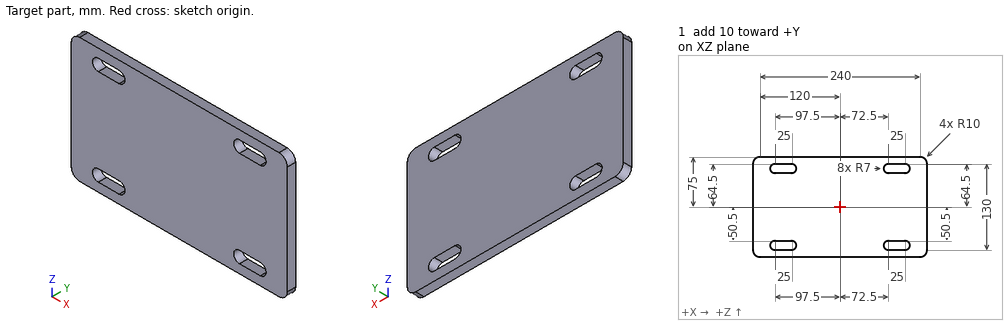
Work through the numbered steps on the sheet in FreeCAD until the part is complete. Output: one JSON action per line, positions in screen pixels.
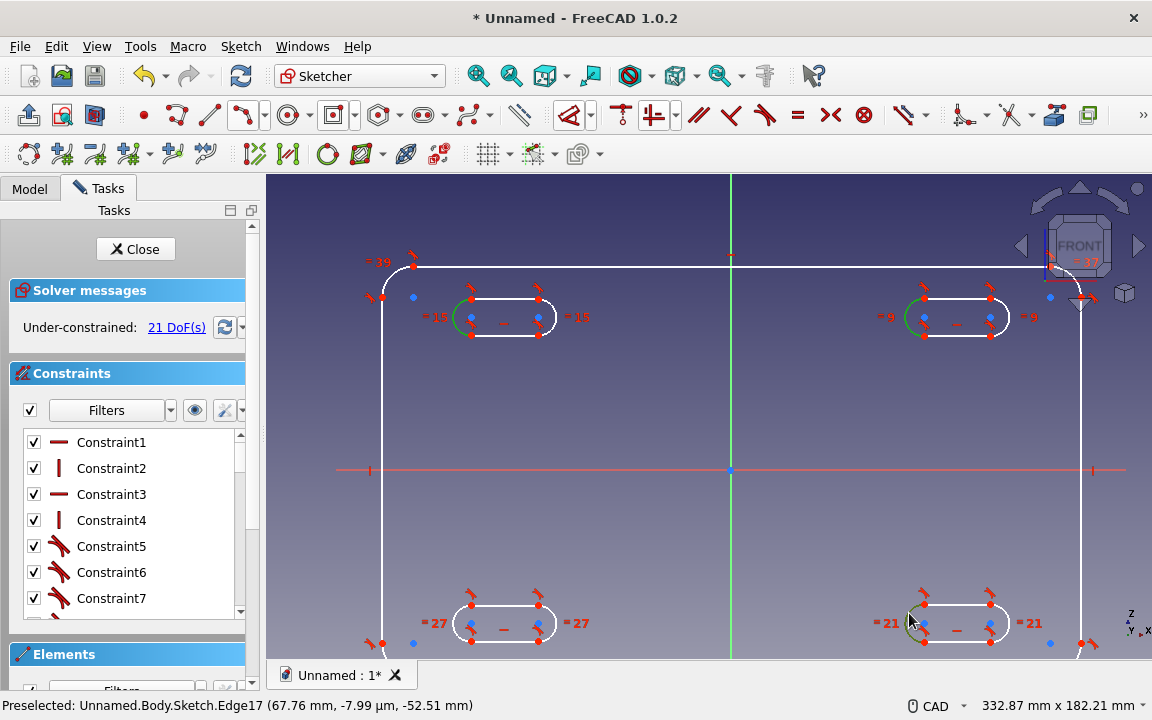
{"action": "left_click", "coordinate": [457, 613]}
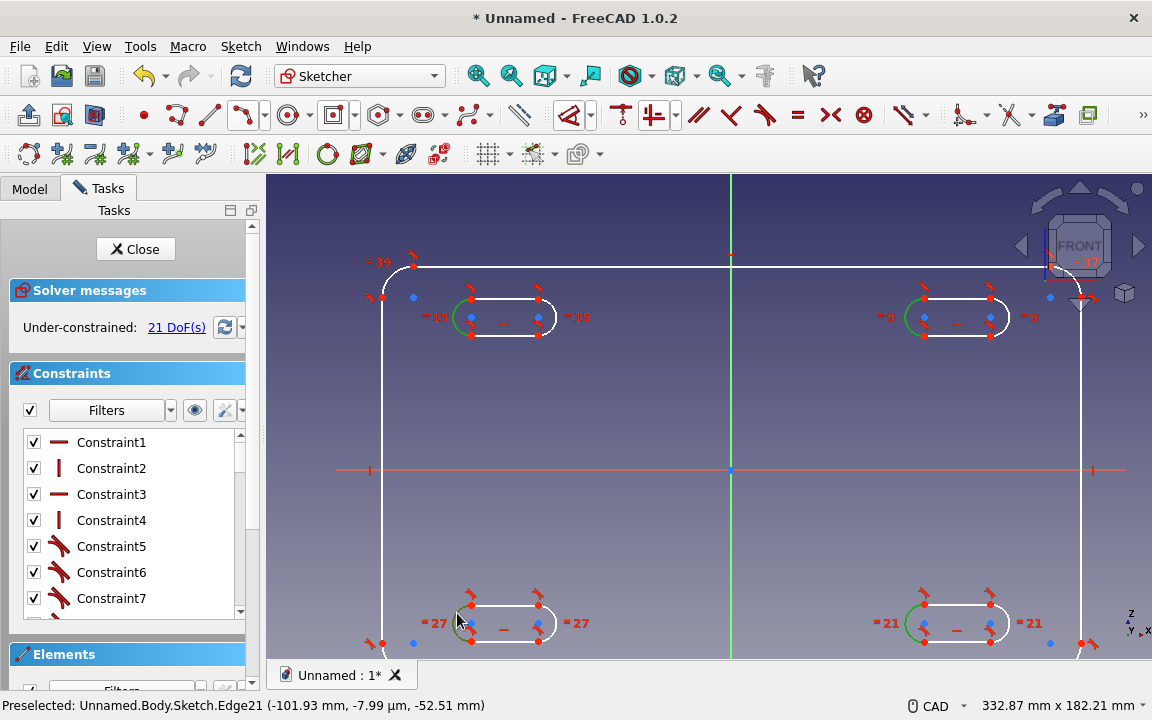
{"action": "left_click", "coordinate": [798, 116]}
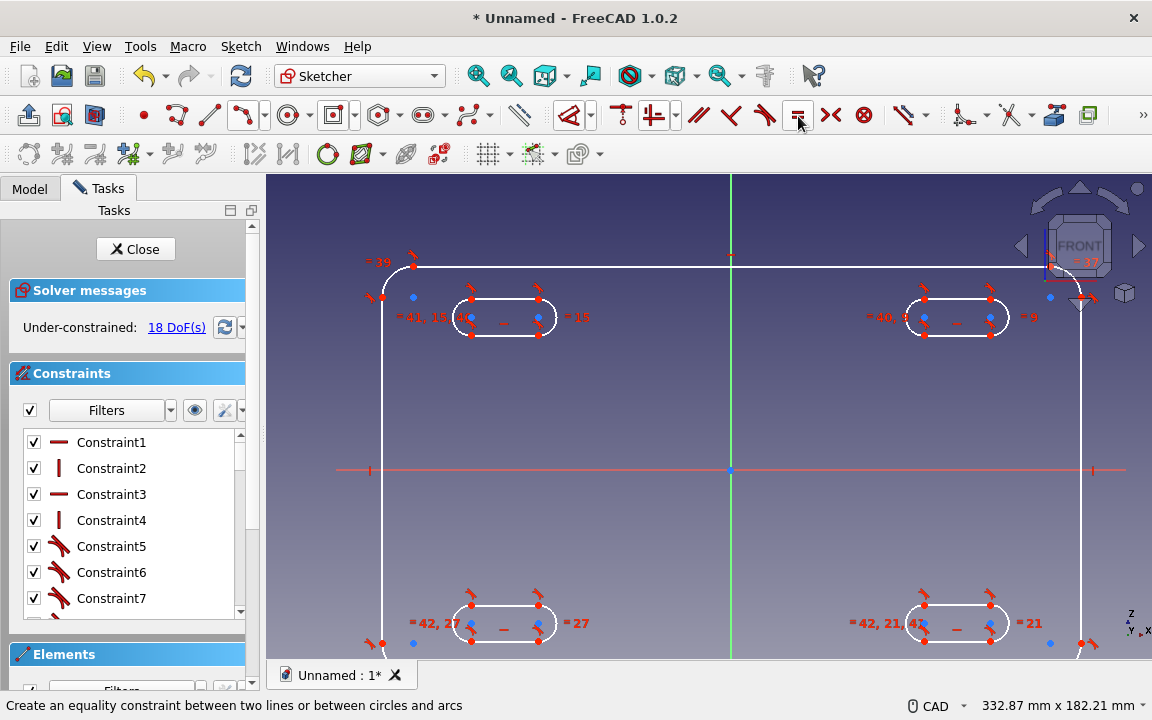
{"action": "left_click", "coordinate": [568, 116]}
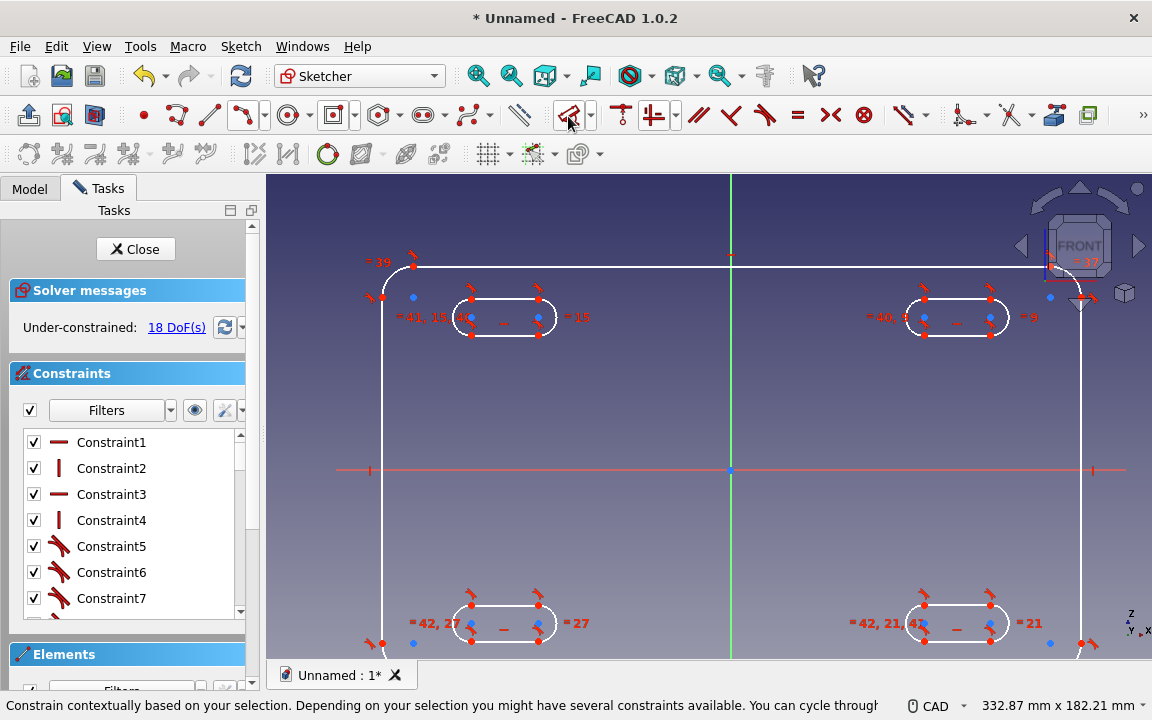
{"action": "scroll", "coordinate": [457, 307], "scroll_direction": "down", "scroll_amount": 2}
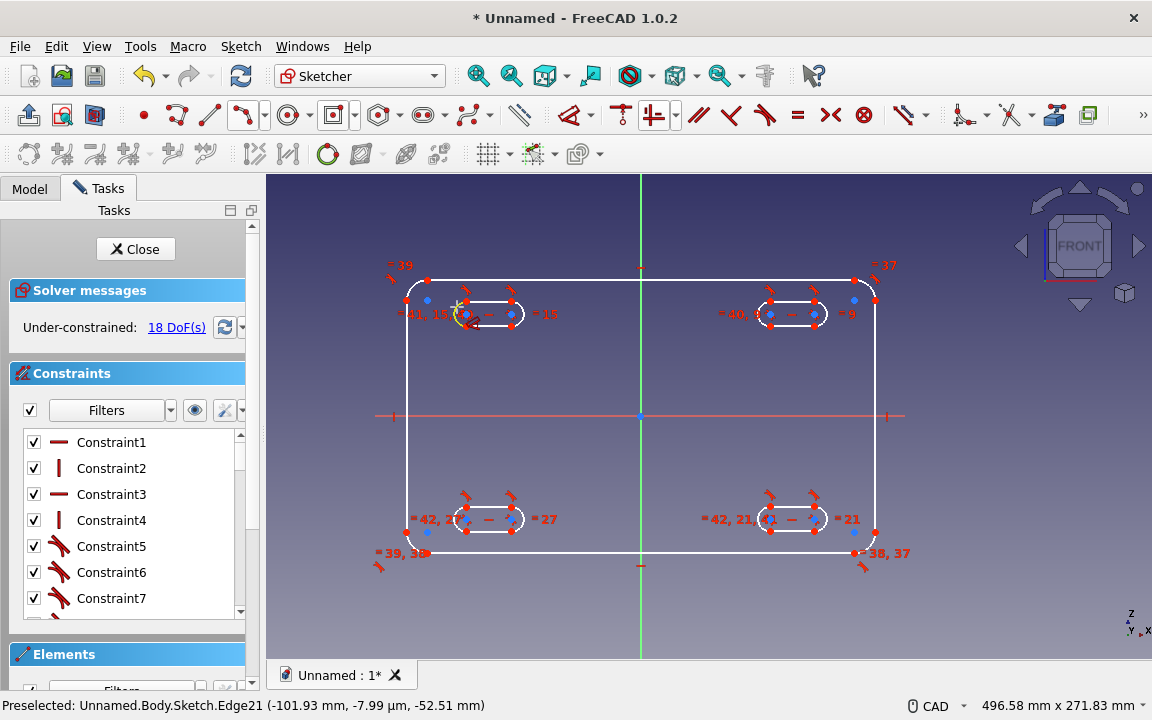
{"action": "scroll", "coordinate": [873, 291], "scroll_direction": "up", "scroll_amount": 4}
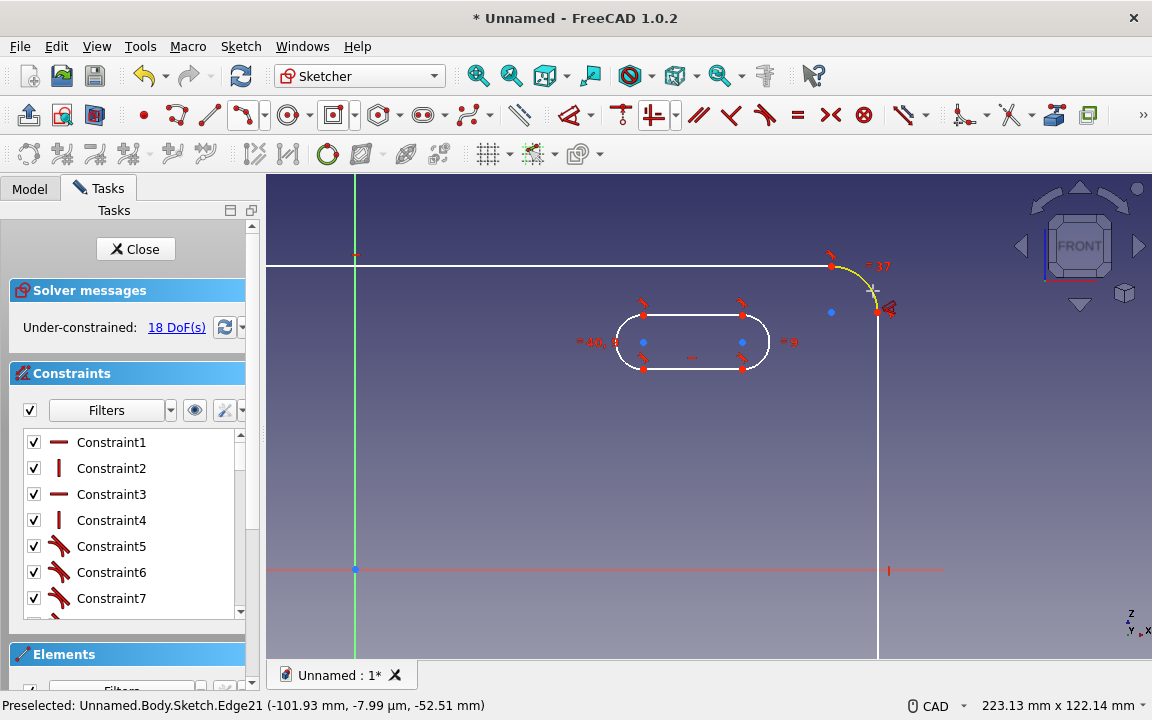
{"action": "left_click", "coordinate": [872, 292]}
{"action": "left_click", "coordinate": [901, 278]}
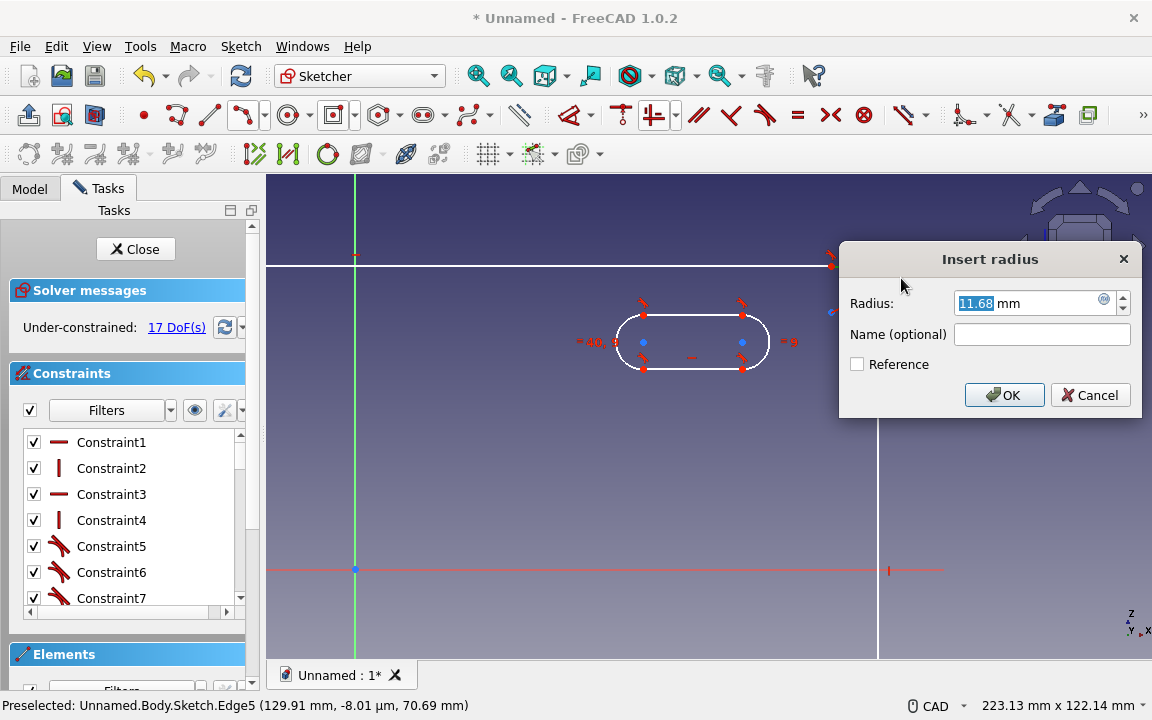
{"action": "type", "text": "10"}
{"action": "key", "text": "Return"}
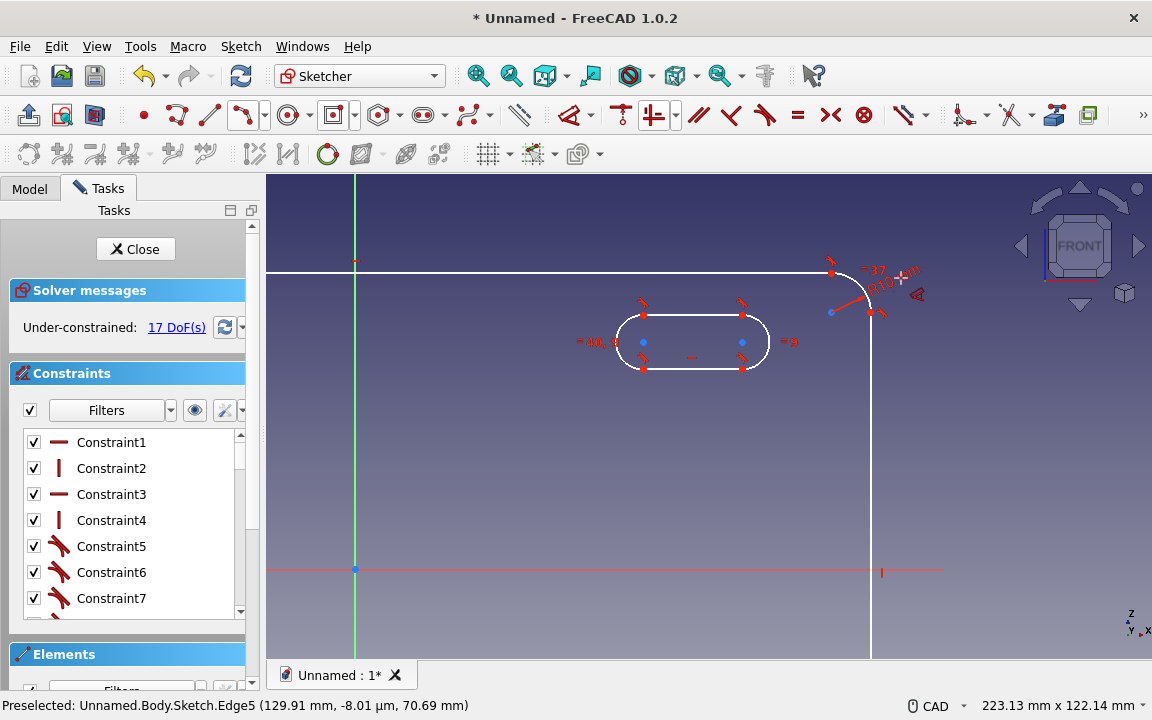
{"action": "scroll", "coordinate": [621, 326], "scroll_direction": "up", "scroll_amount": 2}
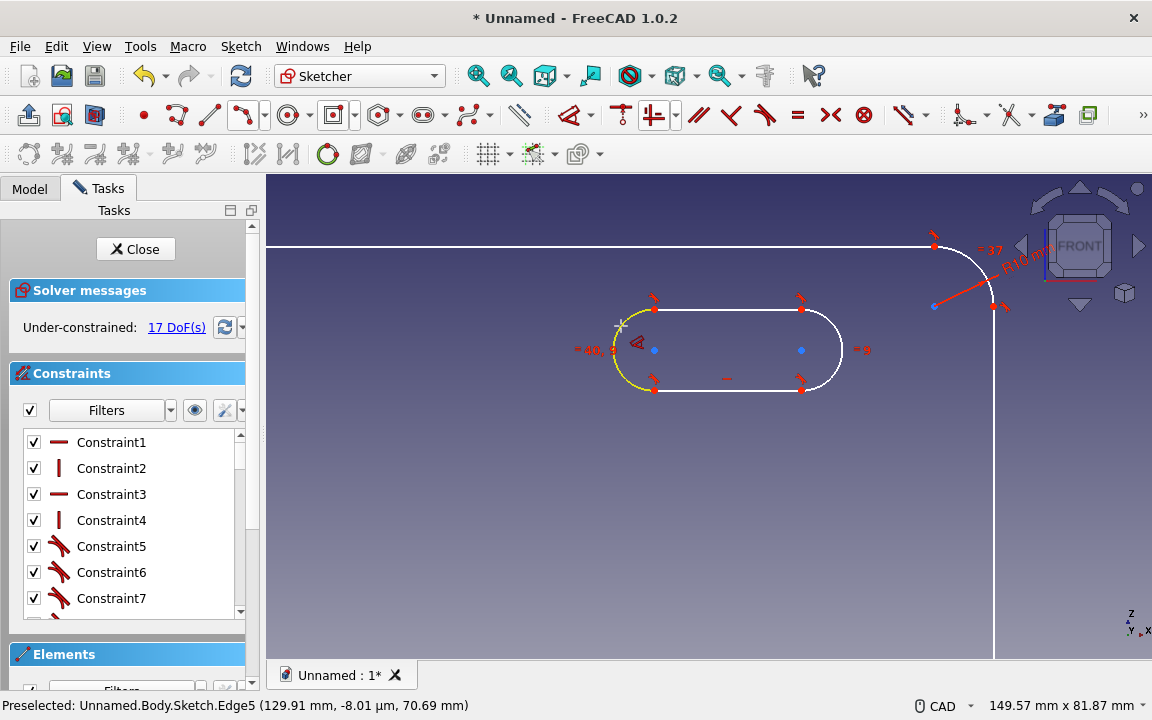
{"action": "left_click", "coordinate": [621, 326]}
{"action": "left_click", "coordinate": [595, 307]}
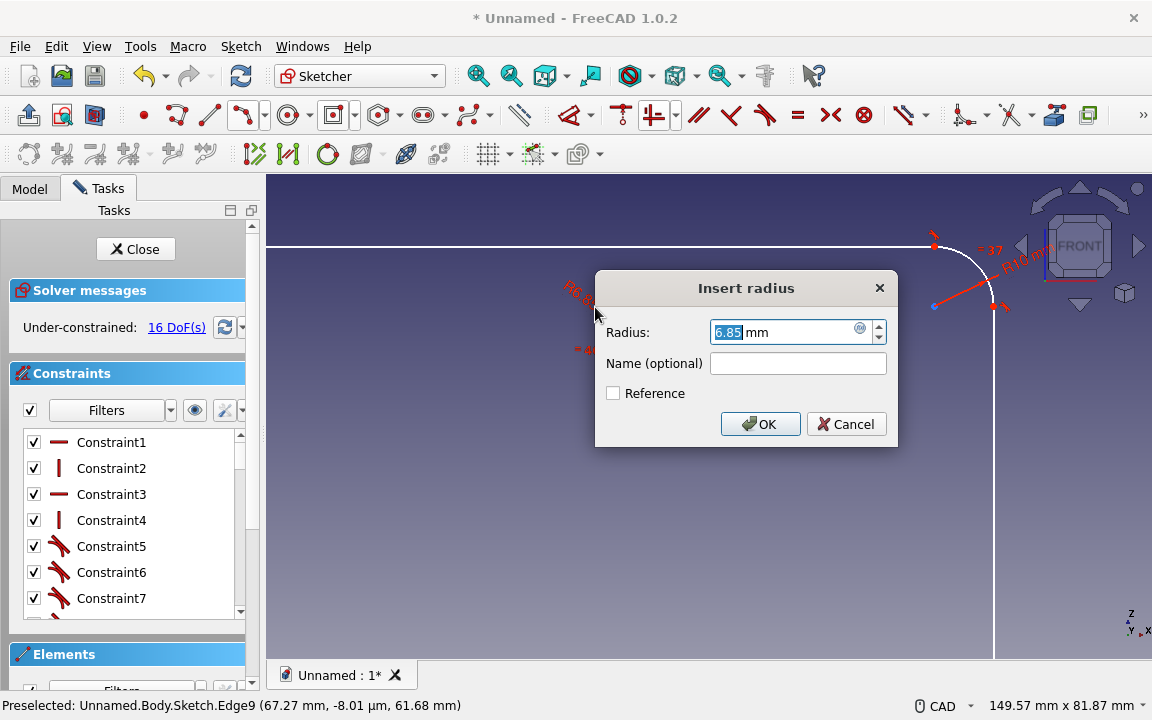
{"action": "type", "text": "7"}
{"action": "key", "text": "Return"}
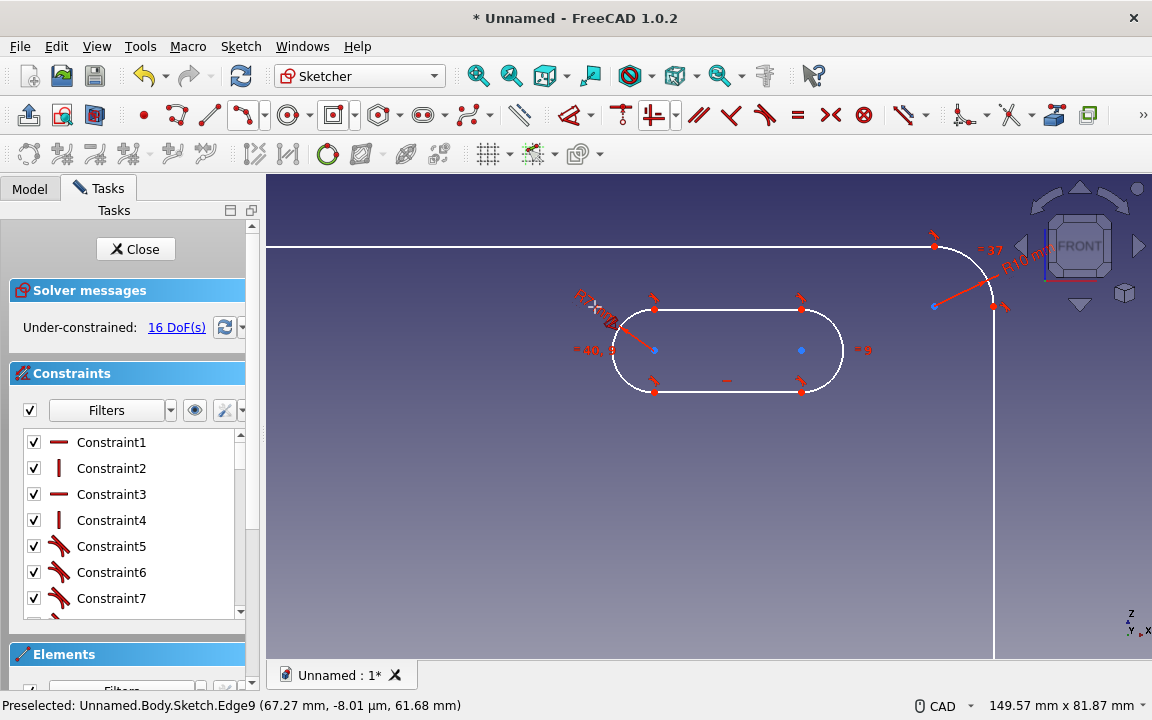
{"action": "left_click", "coordinate": [698, 310]}
{"action": "left_click", "coordinate": [728, 276]}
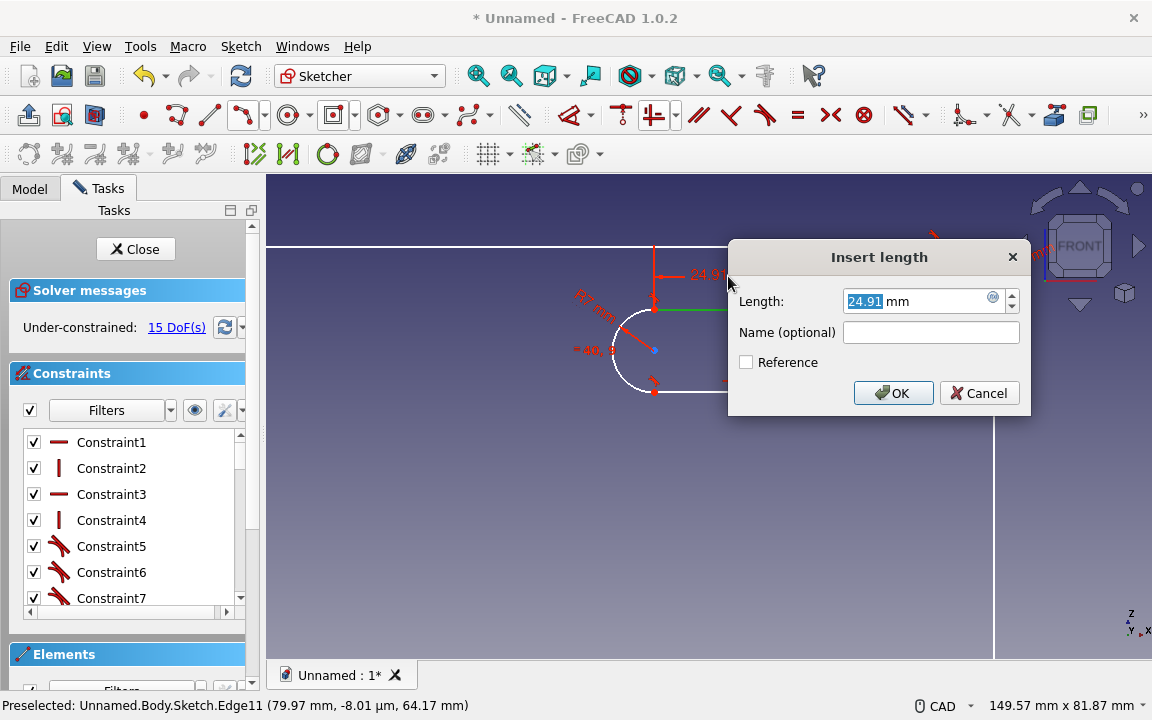
{"action": "type", "text": "25"}
{"action": "key", "text": "Return"}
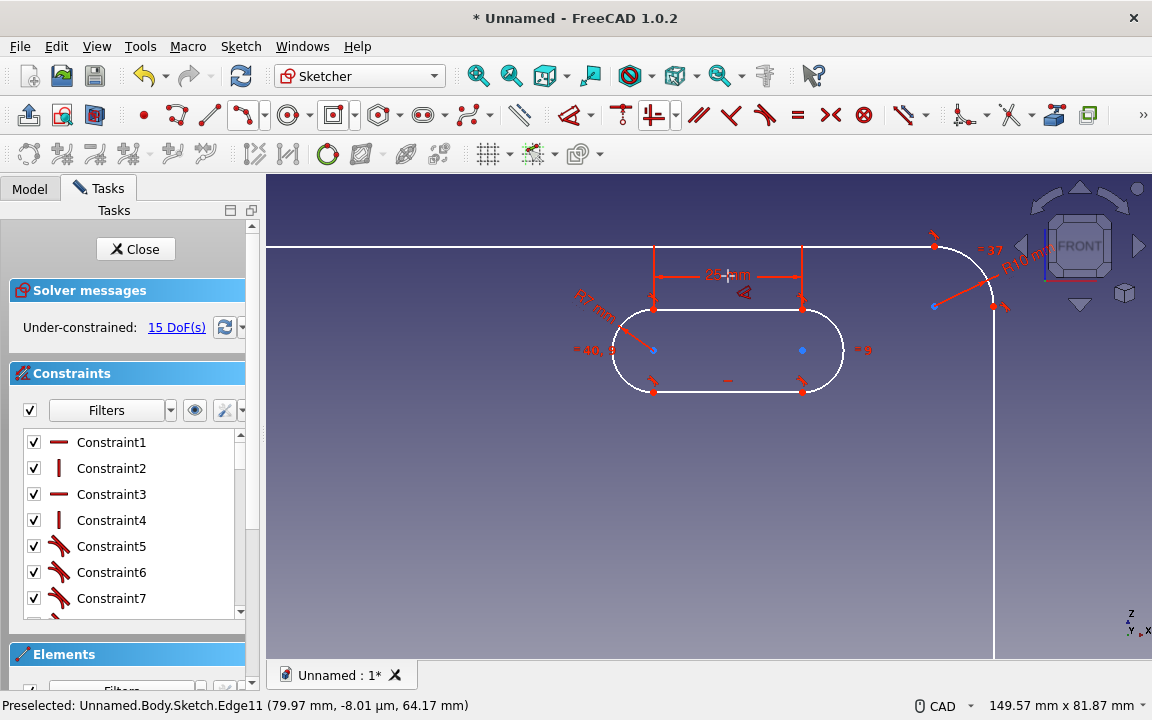
{"action": "scroll", "coordinate": [820, 299], "scroll_direction": "down", "scroll_amount": 6}